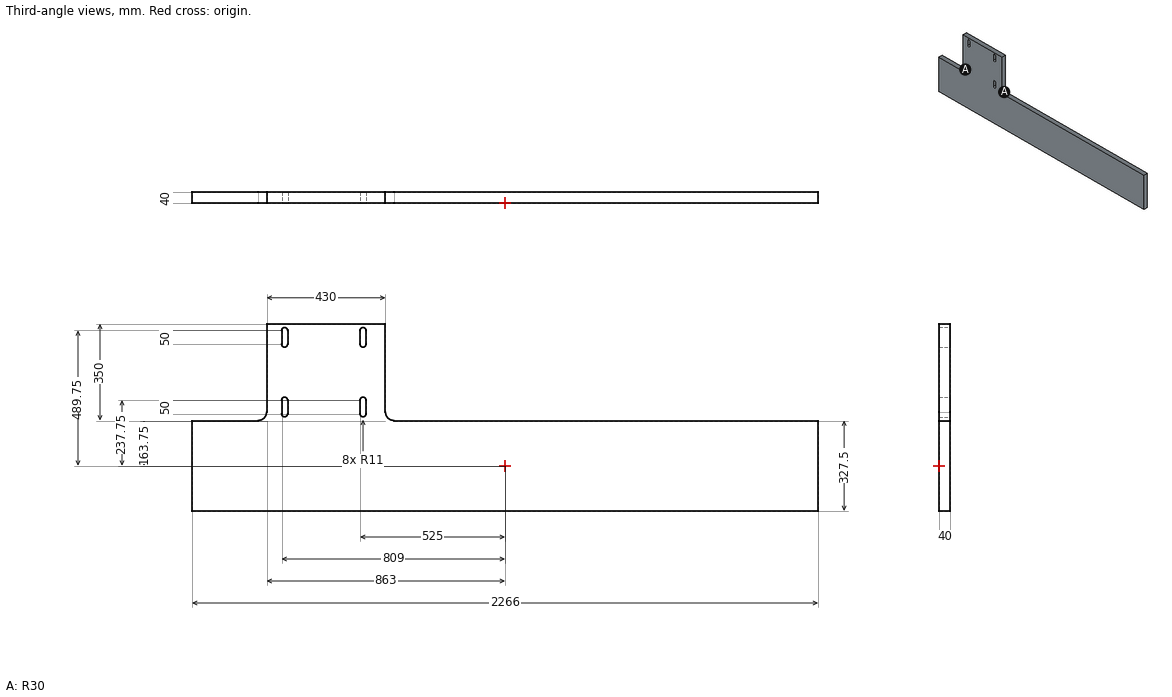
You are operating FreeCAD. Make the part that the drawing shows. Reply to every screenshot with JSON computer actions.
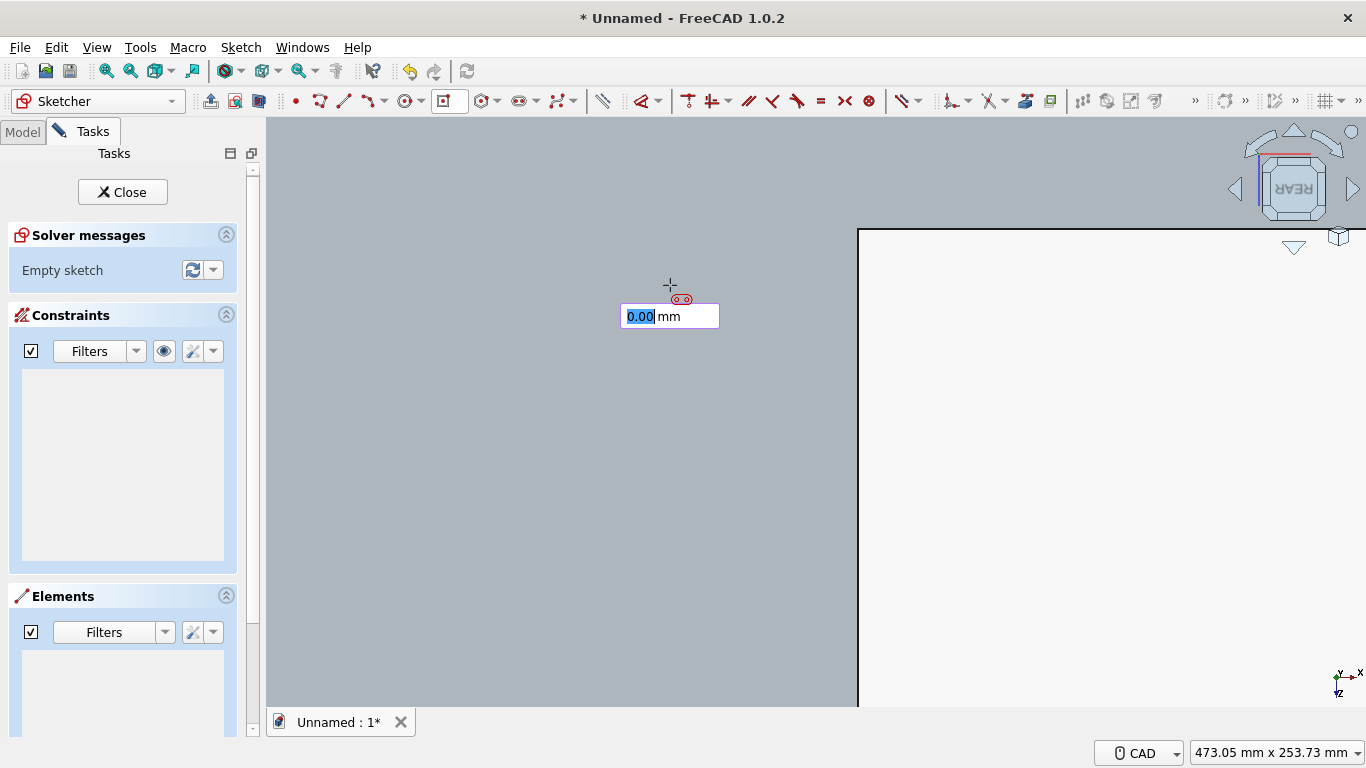
{"action": "left_click", "coordinate": [695, 343]}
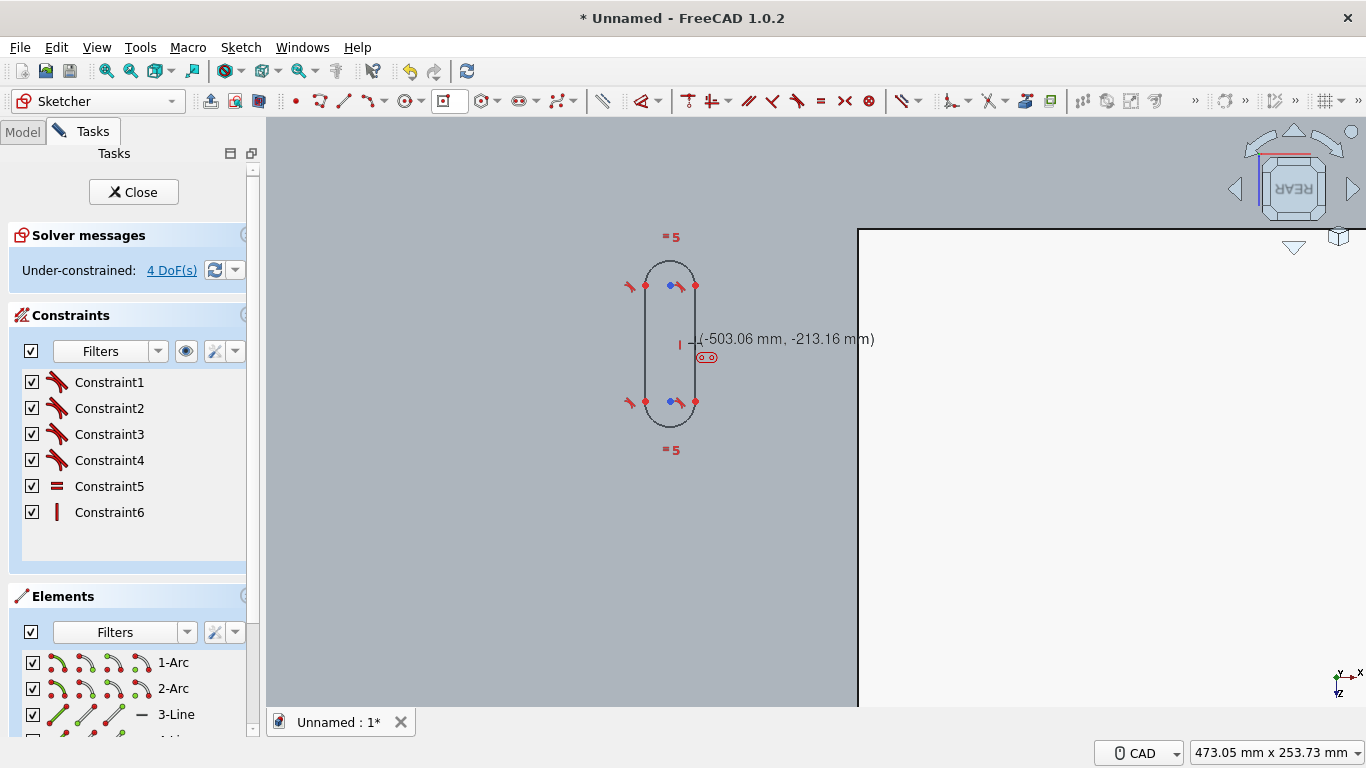
{"action": "scroll", "coordinate": [671, 404], "scroll_direction": "down", "scroll_amount": 6}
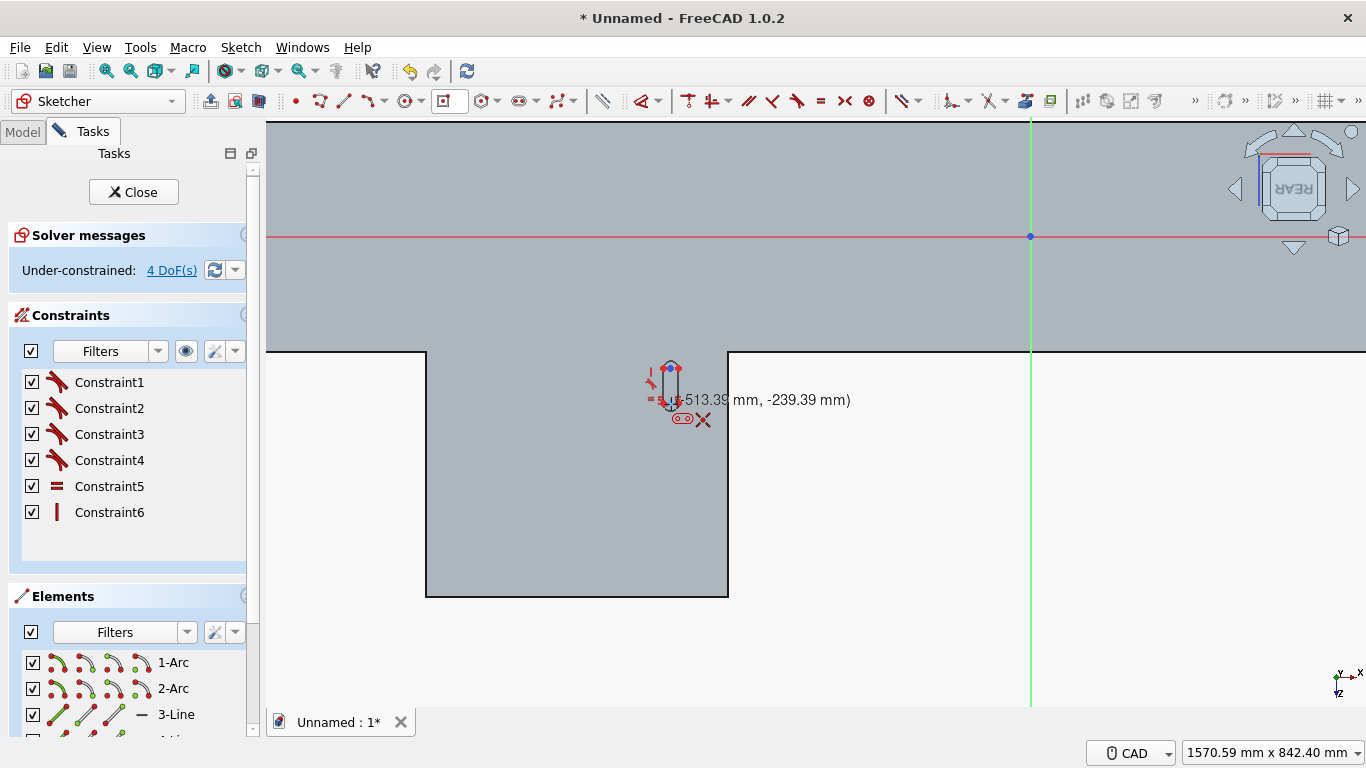
{"action": "scroll", "coordinate": [472, 403], "scroll_direction": "up", "scroll_amount": 6}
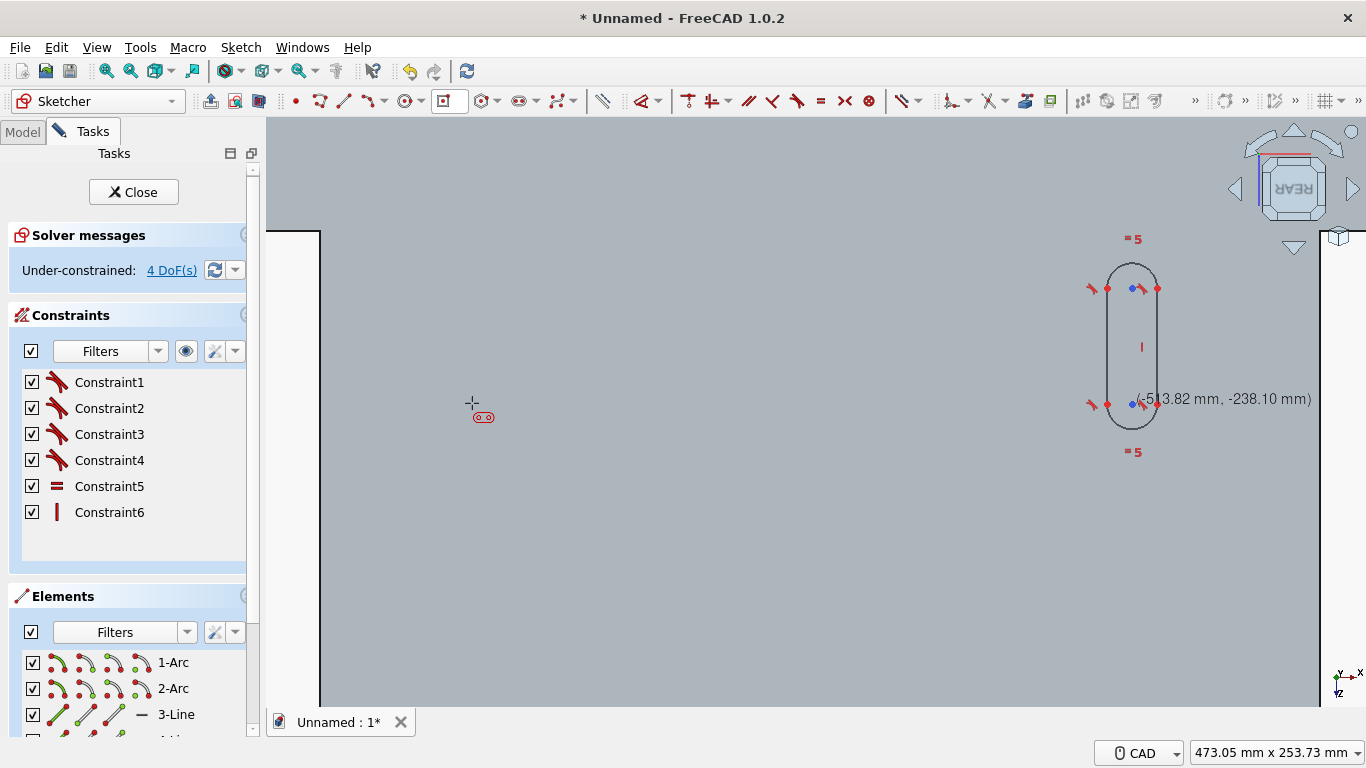
{"action": "left_click", "coordinate": [471, 404]}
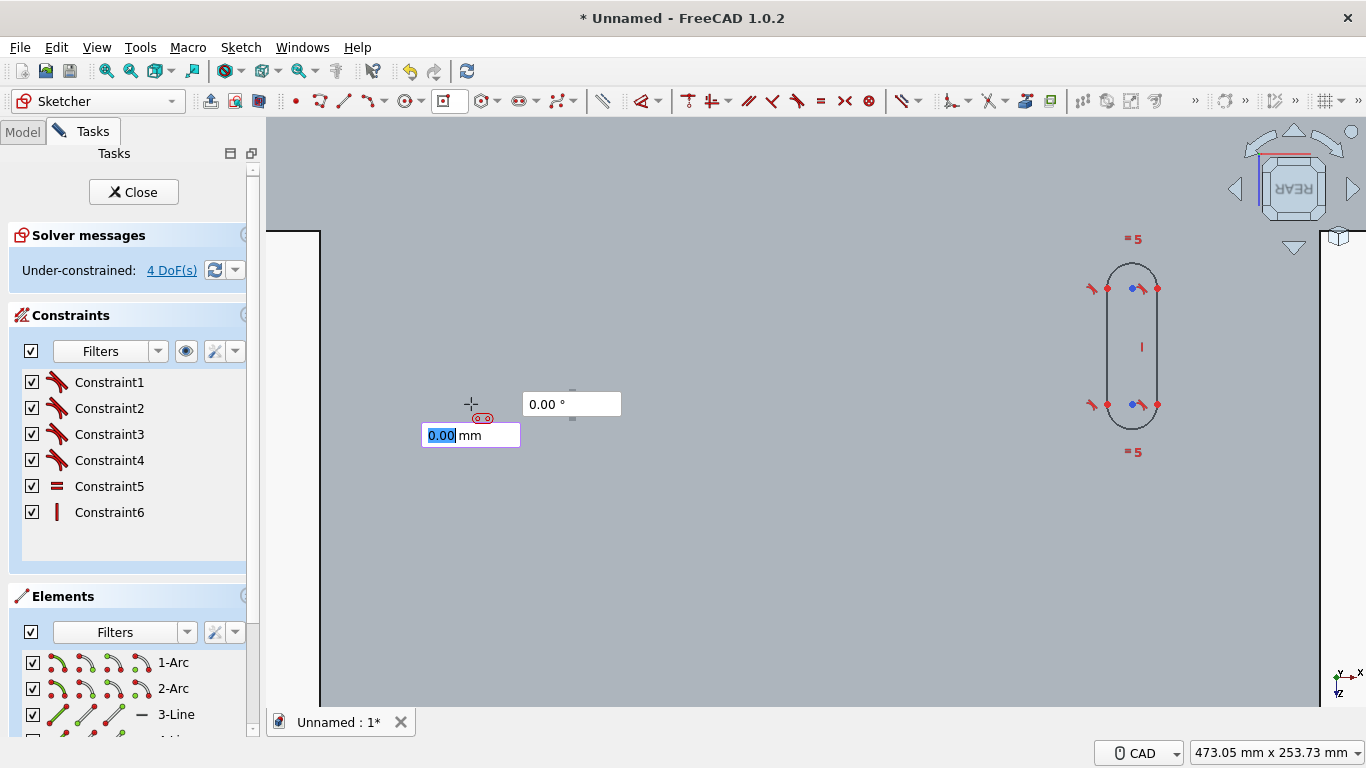
{"action": "left_click", "coordinate": [471, 287]}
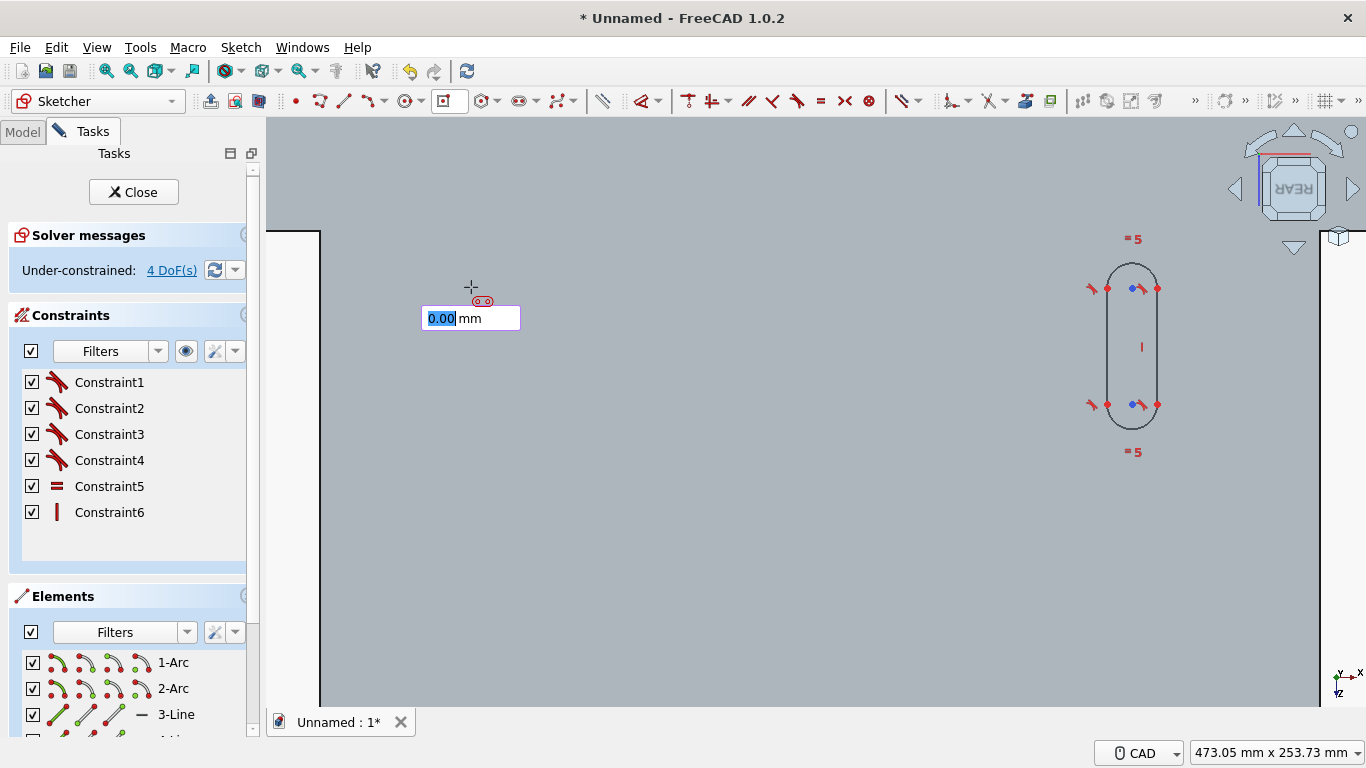
{"action": "left_click", "coordinate": [497, 345]}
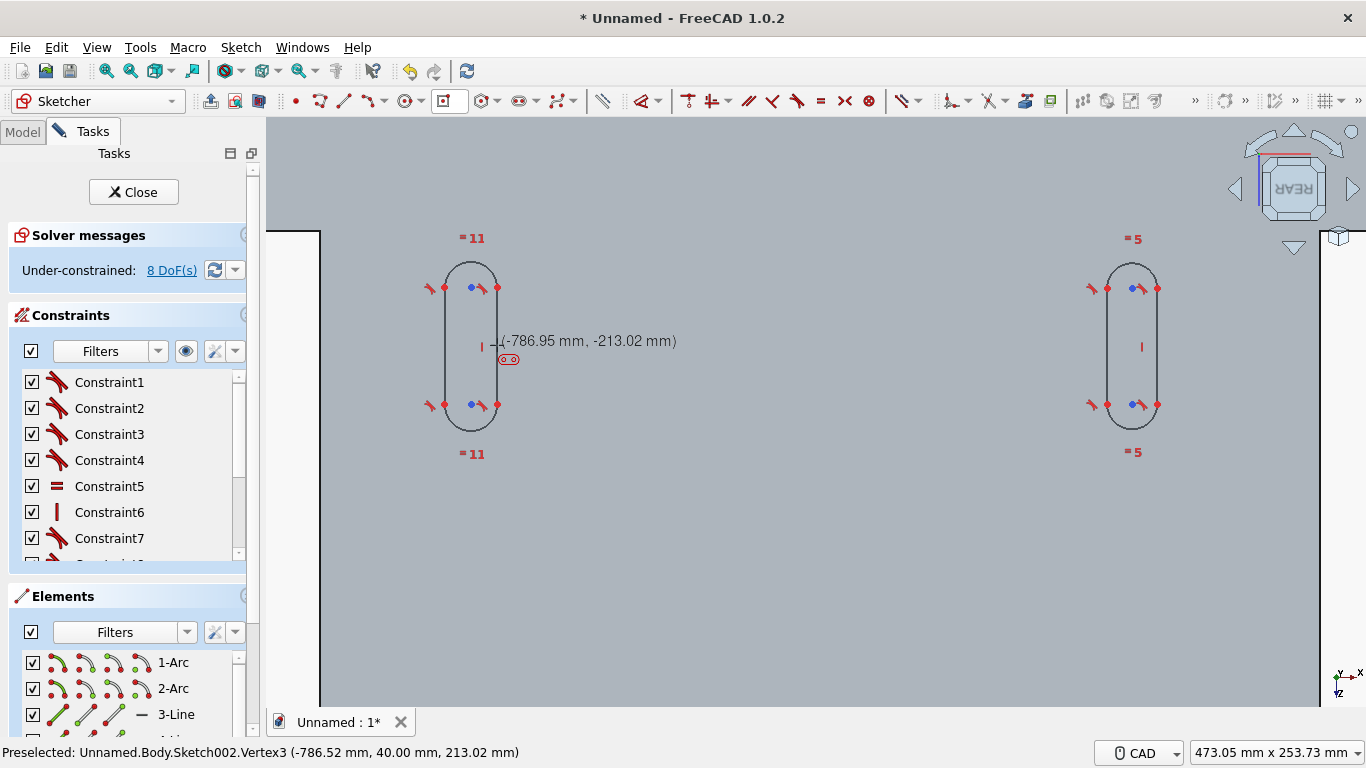
{"action": "scroll", "coordinate": [472, 403], "scroll_direction": "down", "scroll_amount": 6}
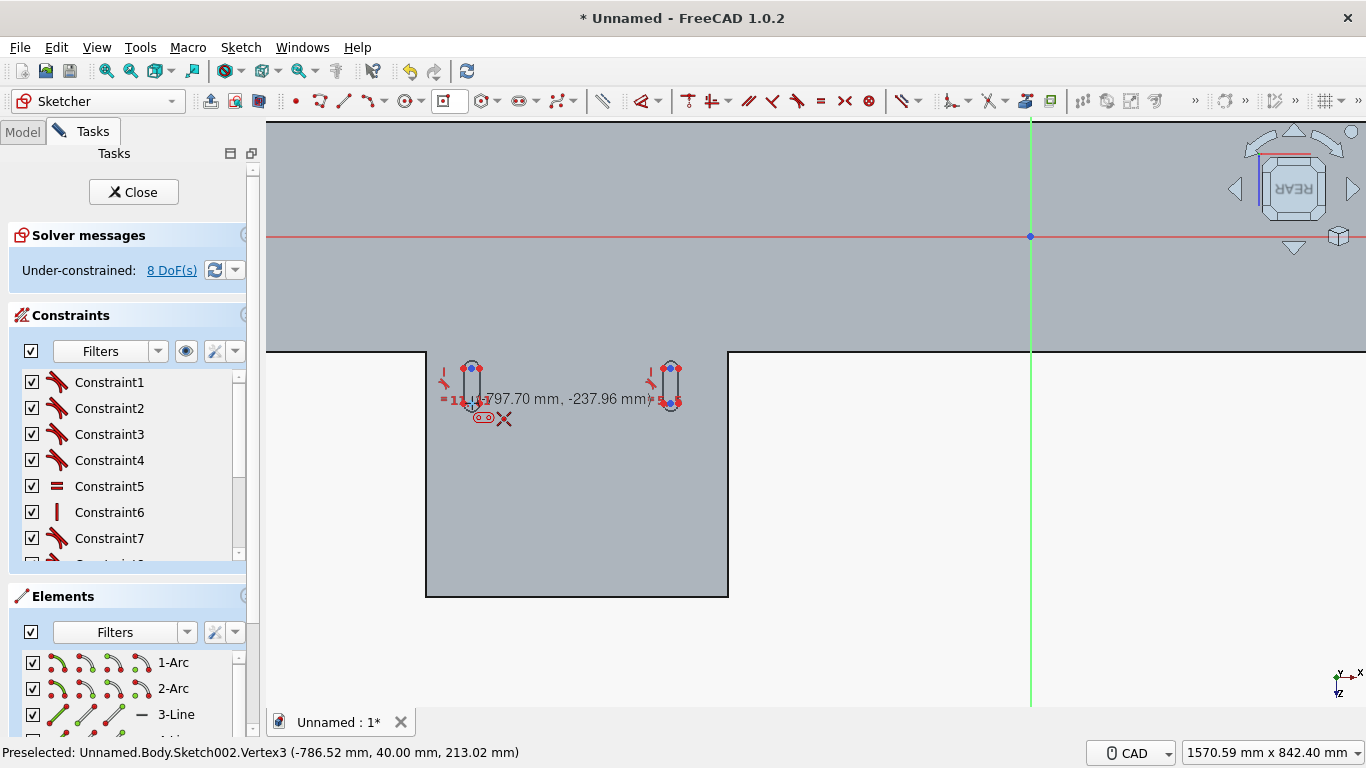
{"action": "scroll", "coordinate": [472, 580], "scroll_direction": "up", "scroll_amount": 6}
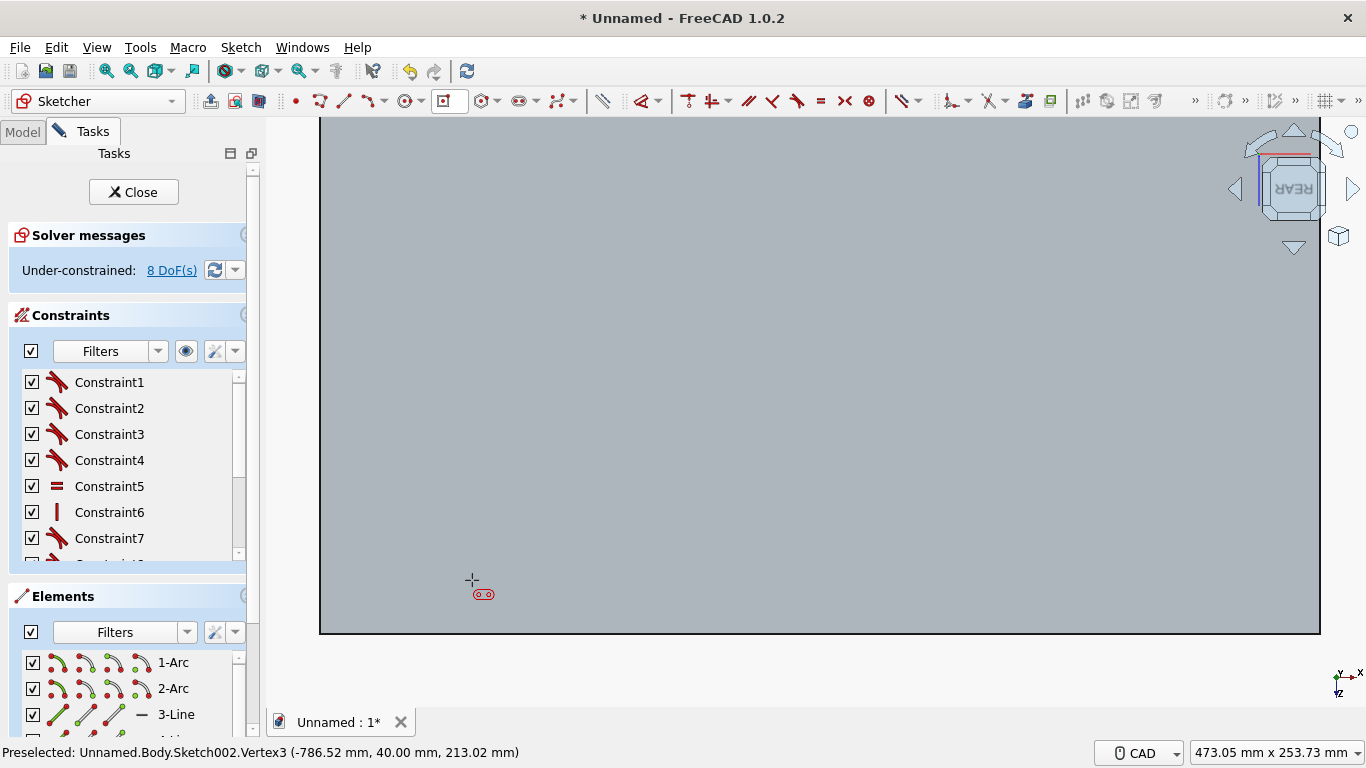
{"action": "left_click", "coordinate": [471, 578]}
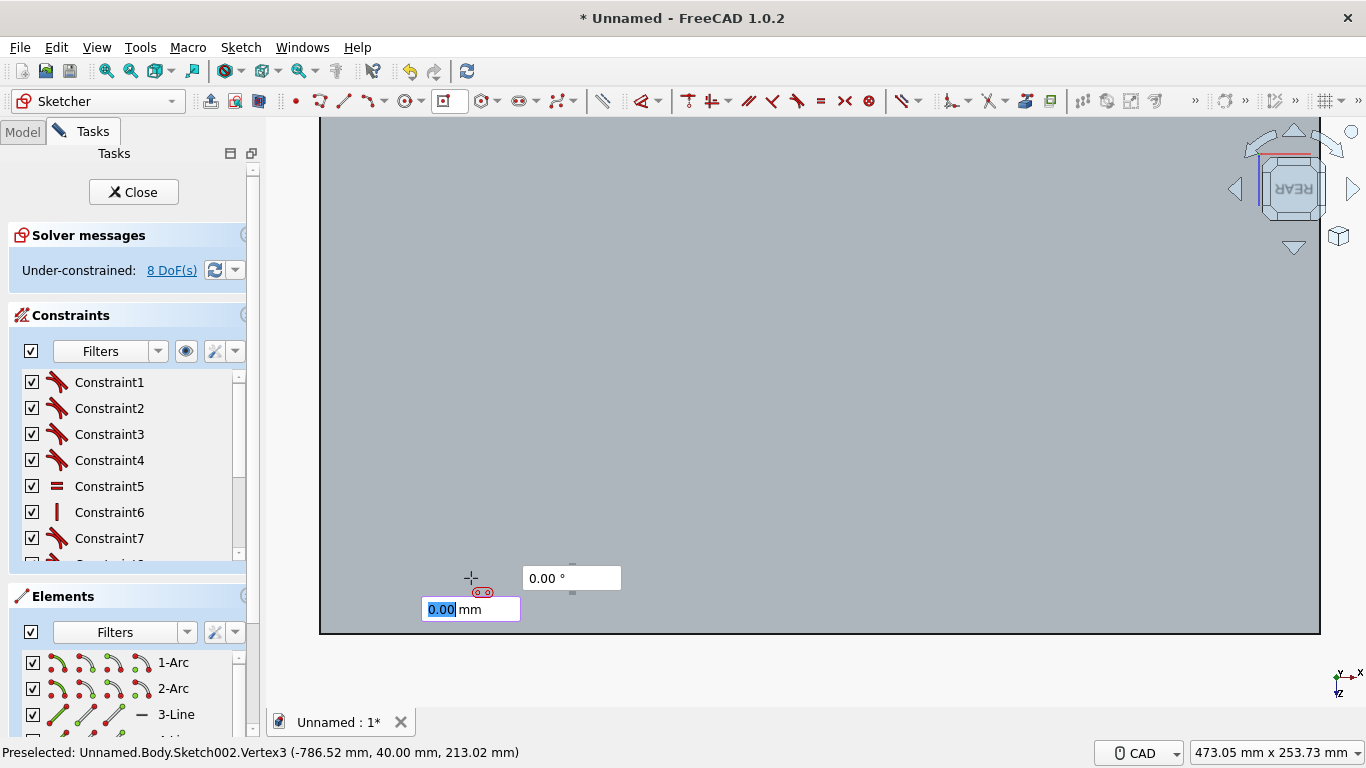
{"action": "left_click", "coordinate": [471, 462]}